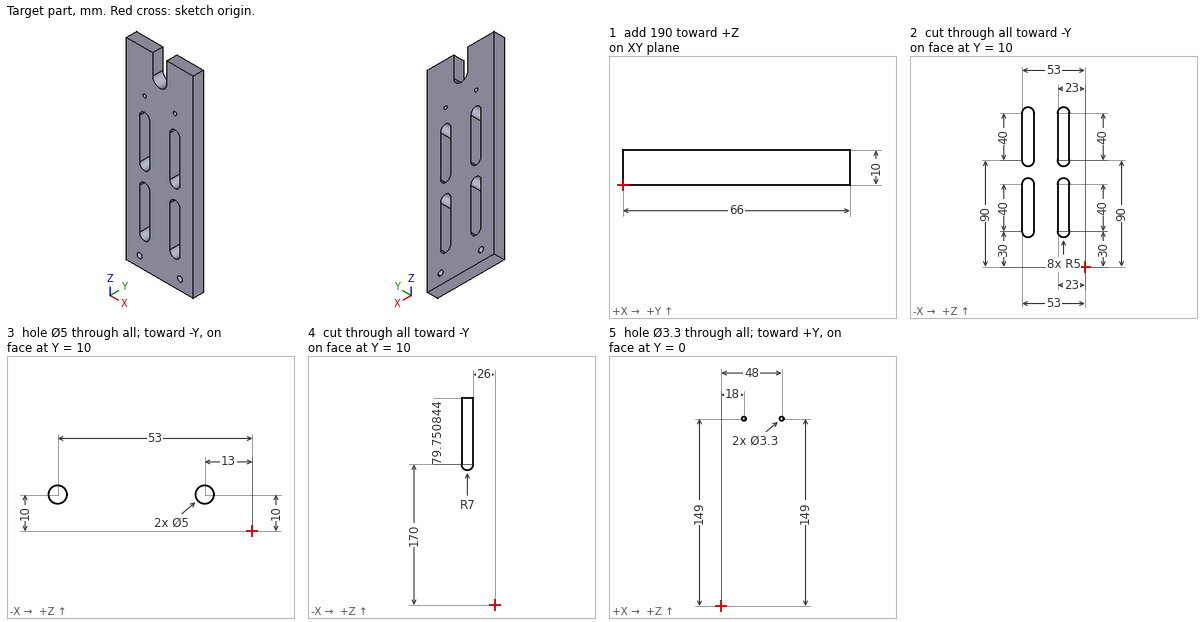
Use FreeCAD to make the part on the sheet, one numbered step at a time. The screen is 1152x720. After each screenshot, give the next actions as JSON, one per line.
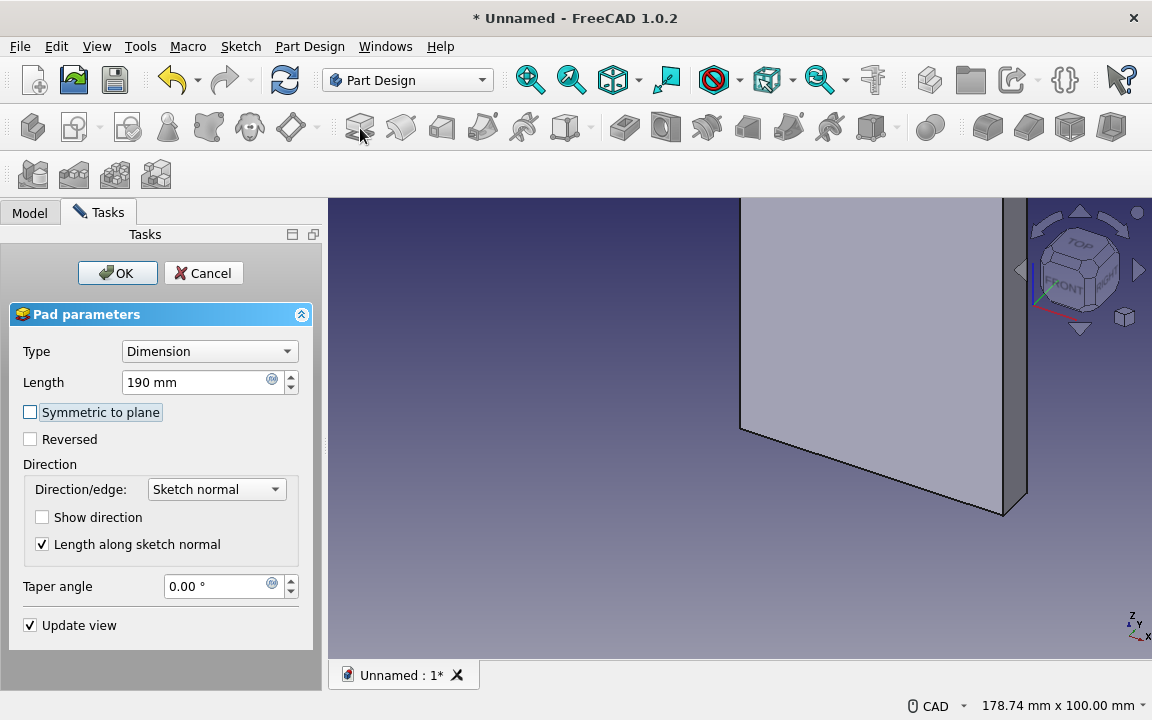
{"action": "left_click", "coordinate": [118, 273]}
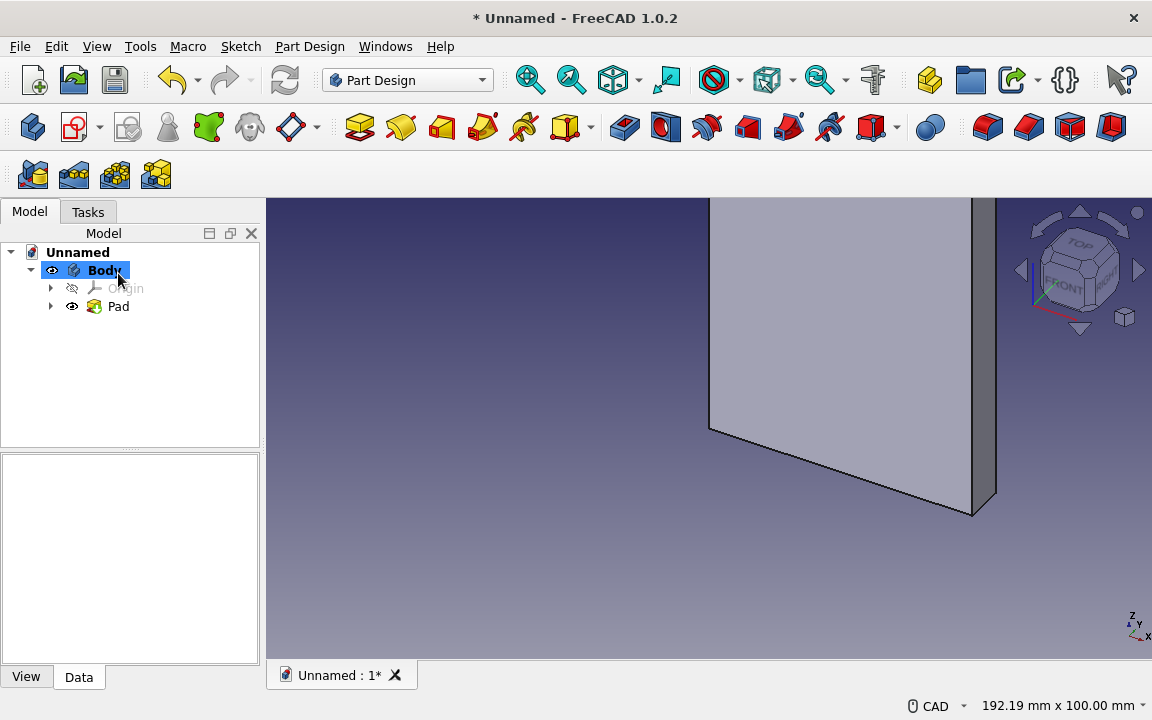
{"action": "left_click", "coordinate": [531, 80]}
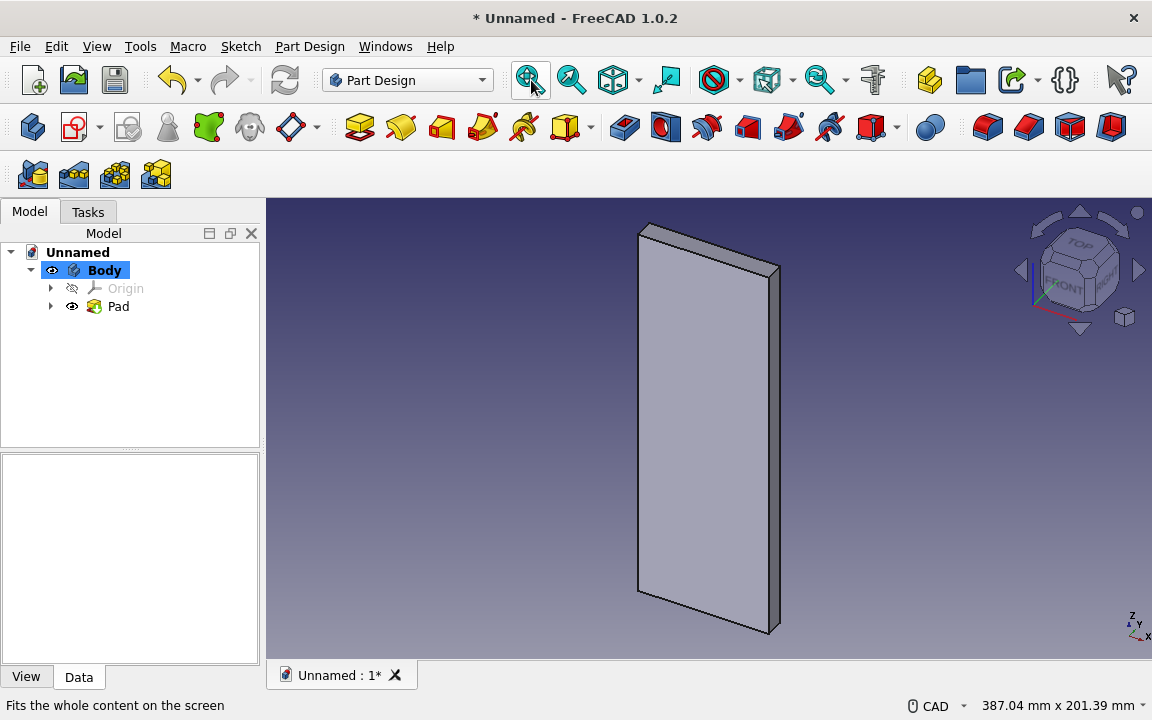
{"action": "key", "text": "4"}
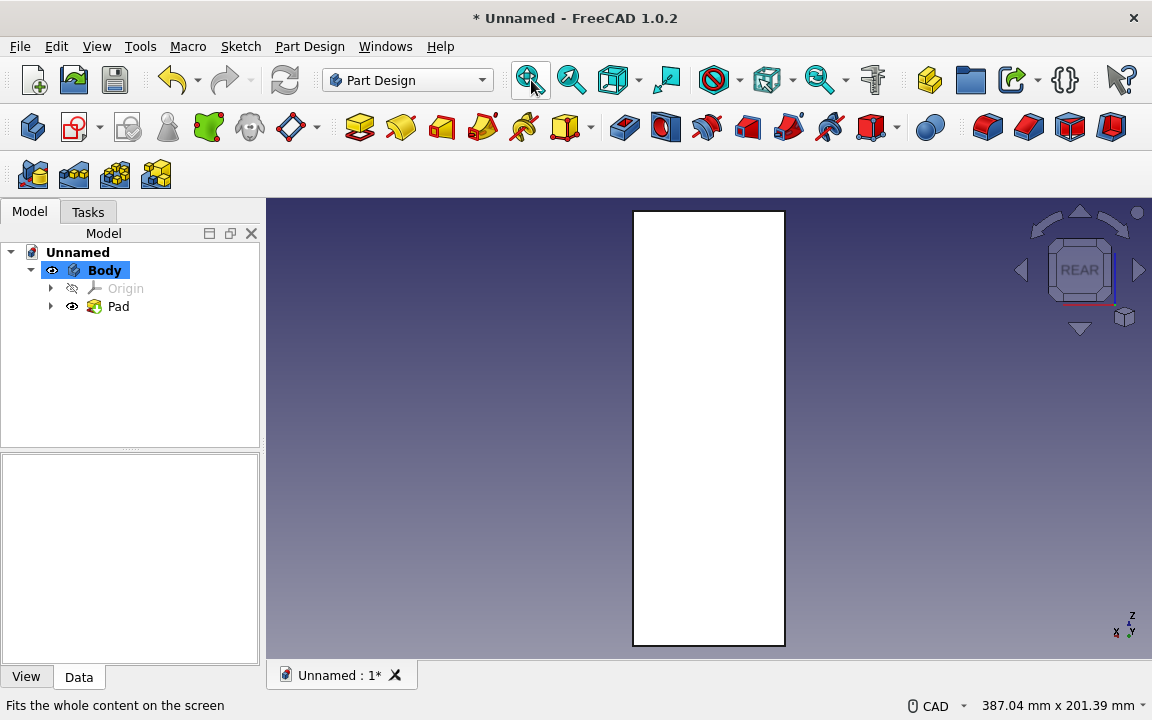
{"action": "left_click", "coordinate": [709, 303]}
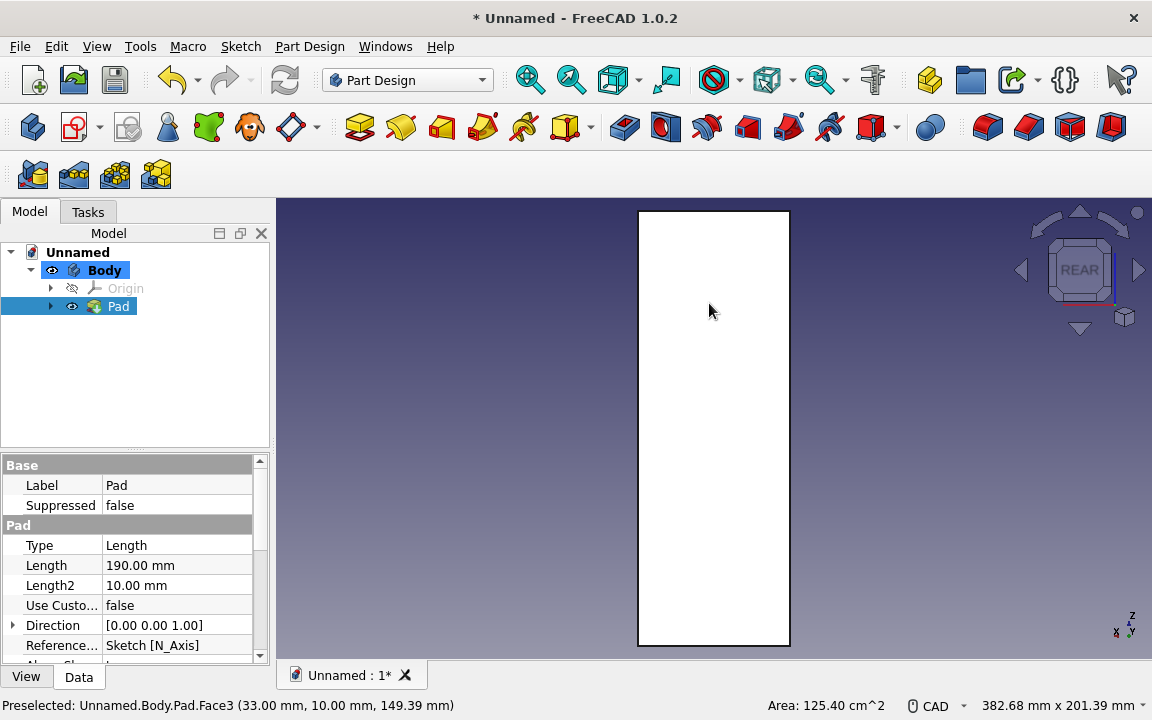
{"action": "left_click", "coordinate": [74, 128]}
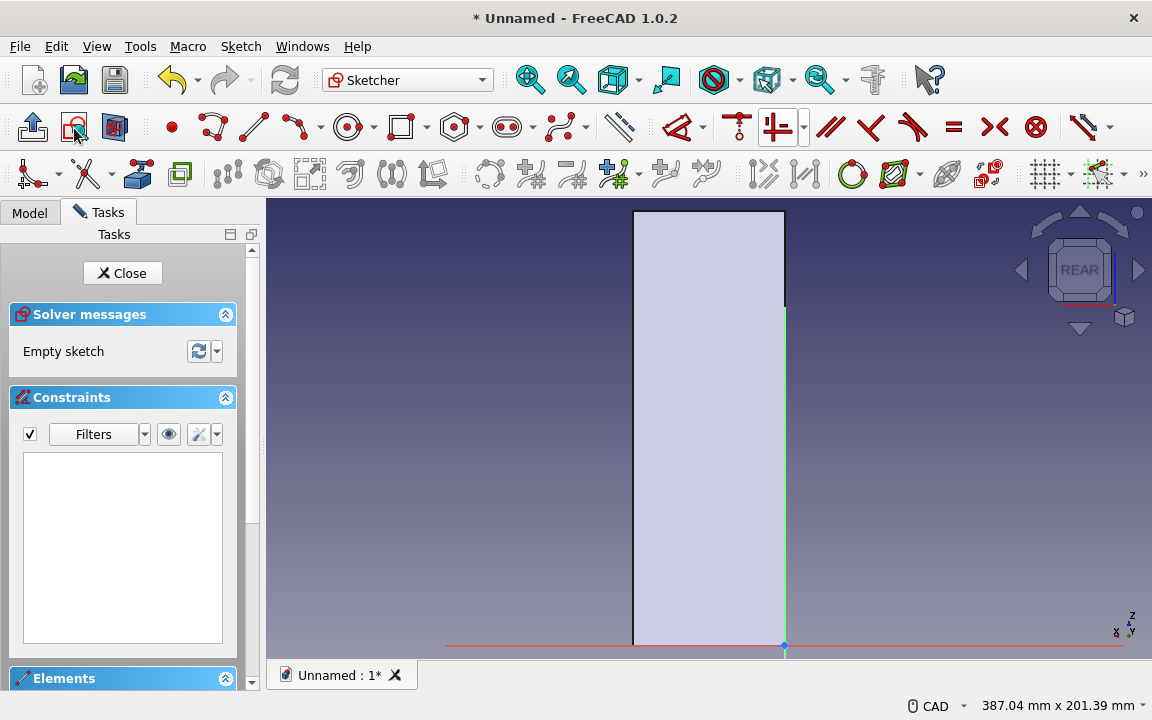
{"action": "scroll", "coordinate": [294, 226], "scroll_direction": "down", "scroll_amount": 1}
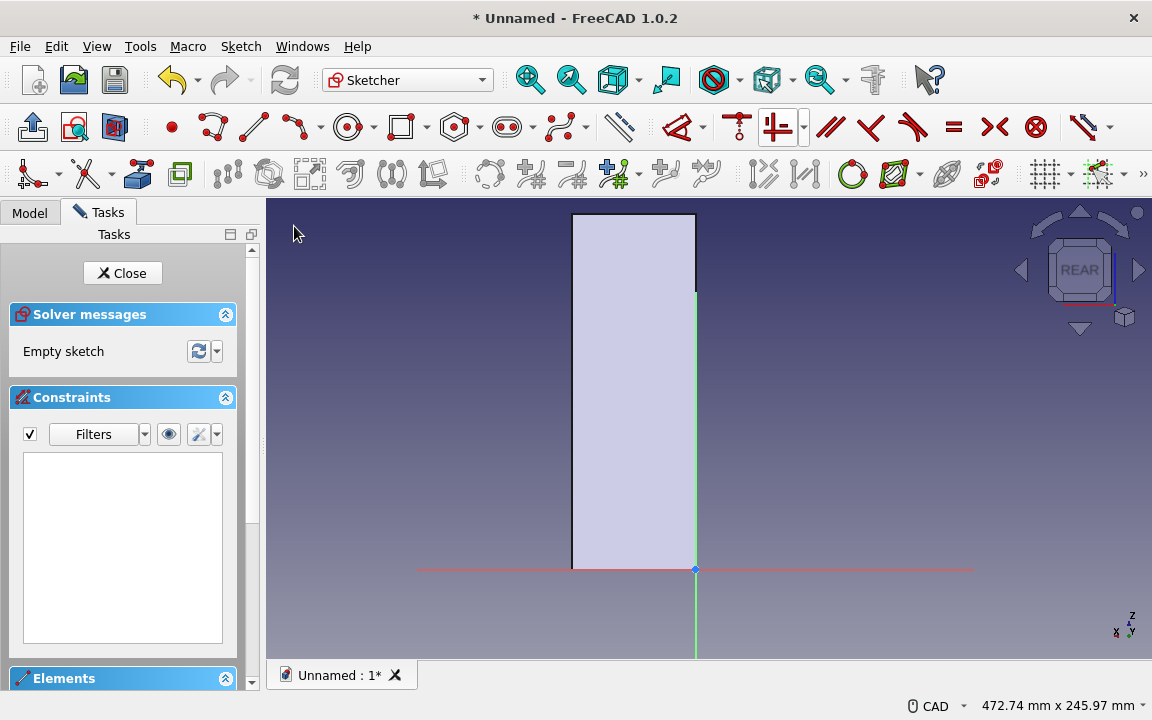
{"action": "left_click", "coordinate": [506, 128]}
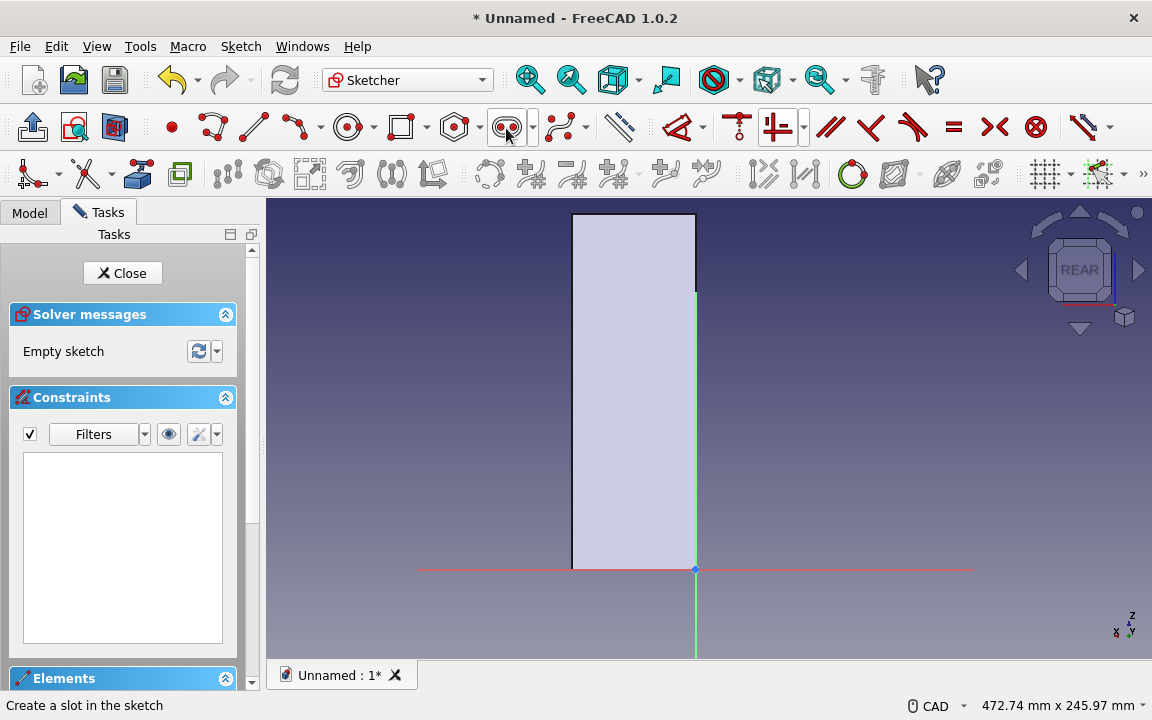
{"action": "scroll", "coordinate": [606, 514], "scroll_direction": "up", "scroll_amount": 5}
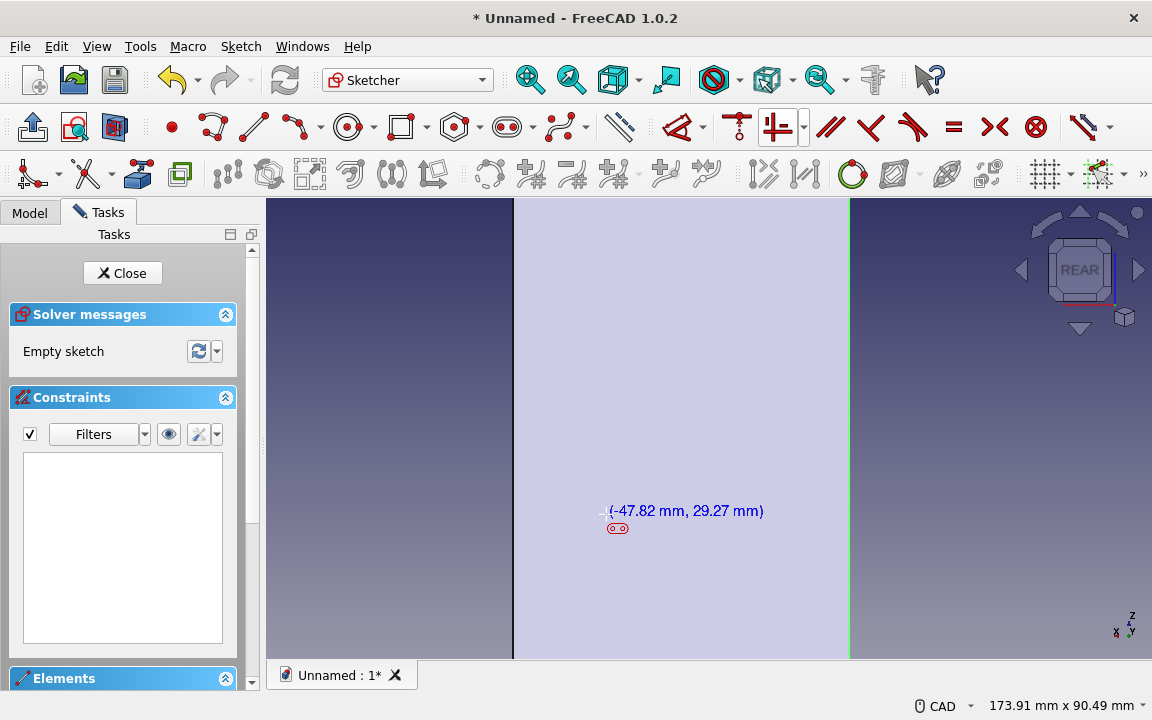
{"action": "left_click", "coordinate": [604, 512]}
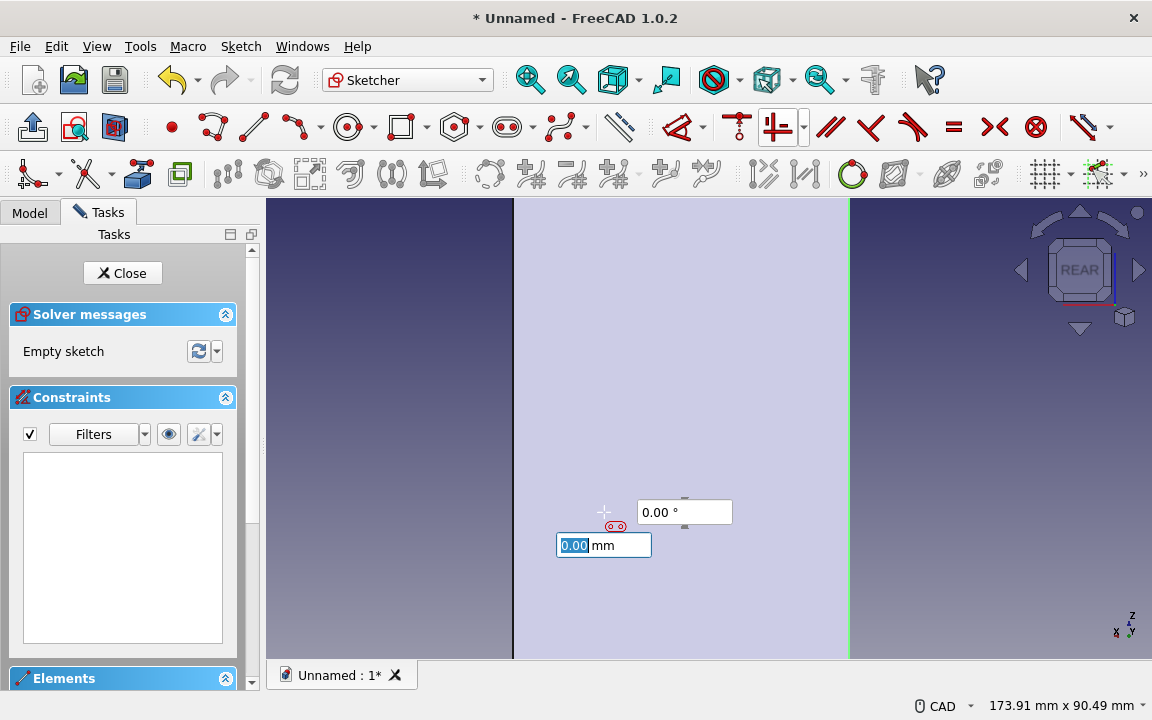
{"action": "left_click", "coordinate": [604, 308]}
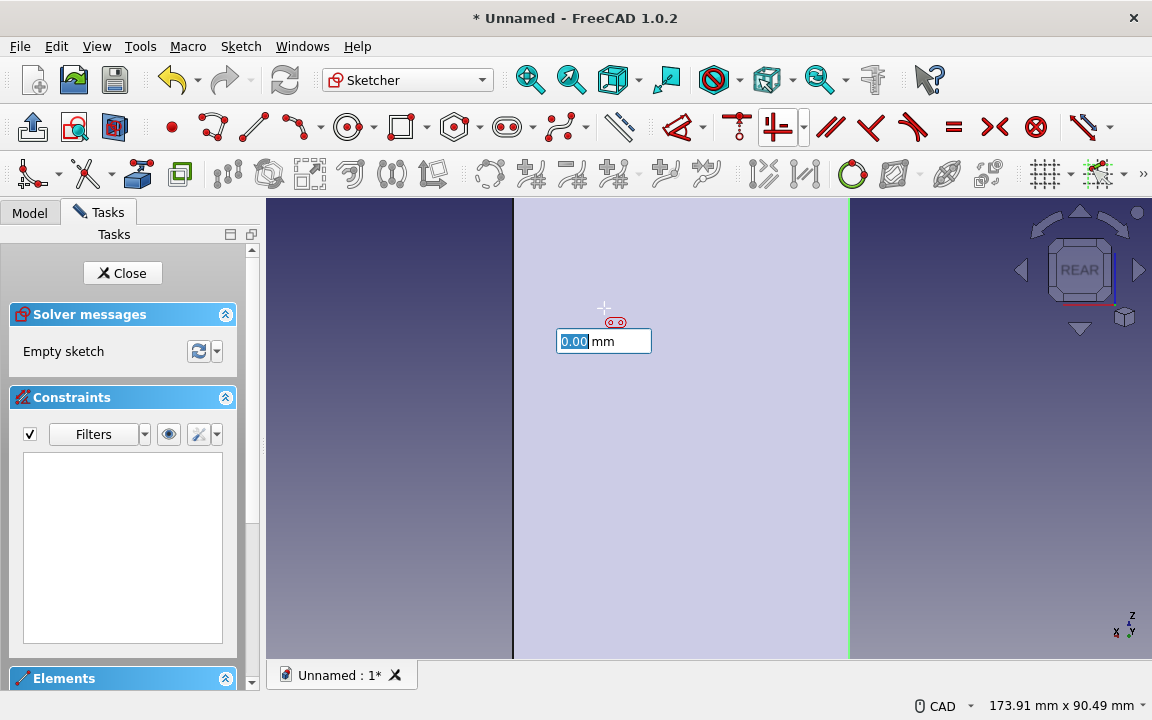
{"action": "left_click", "coordinate": [630, 410]}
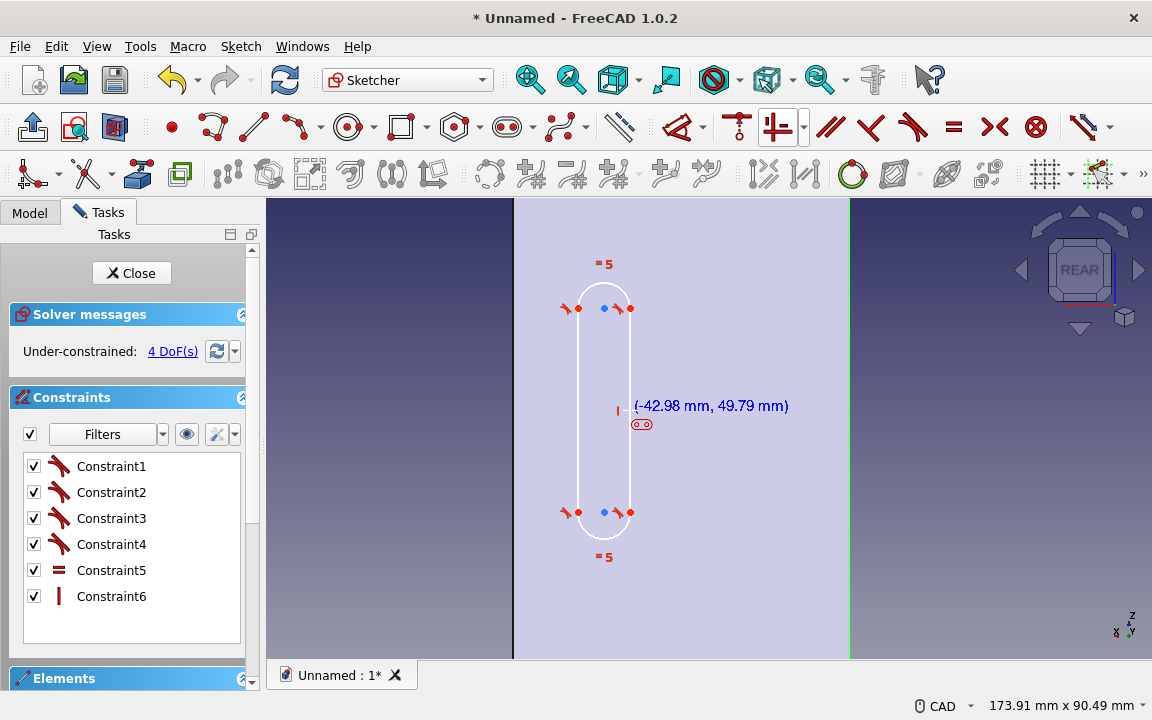
{"action": "left_click", "coordinate": [757, 512]}